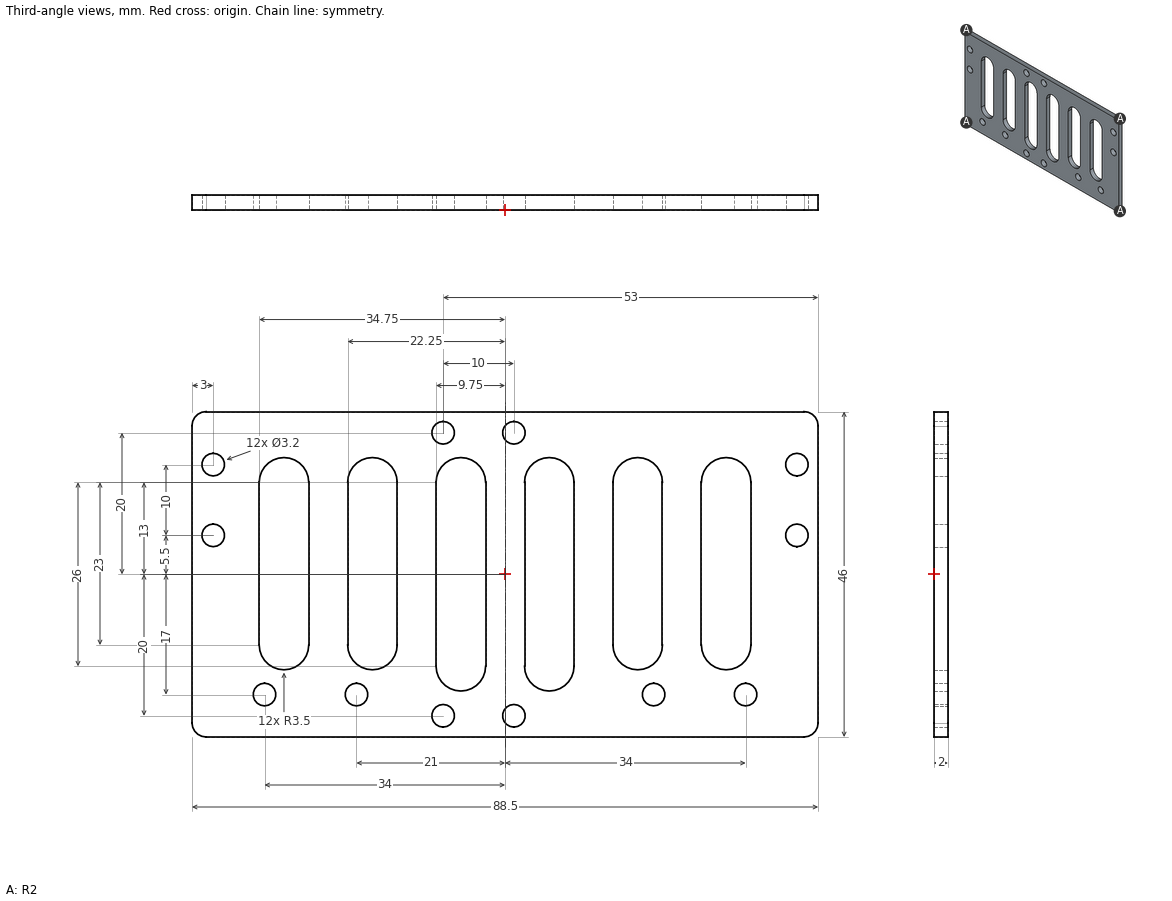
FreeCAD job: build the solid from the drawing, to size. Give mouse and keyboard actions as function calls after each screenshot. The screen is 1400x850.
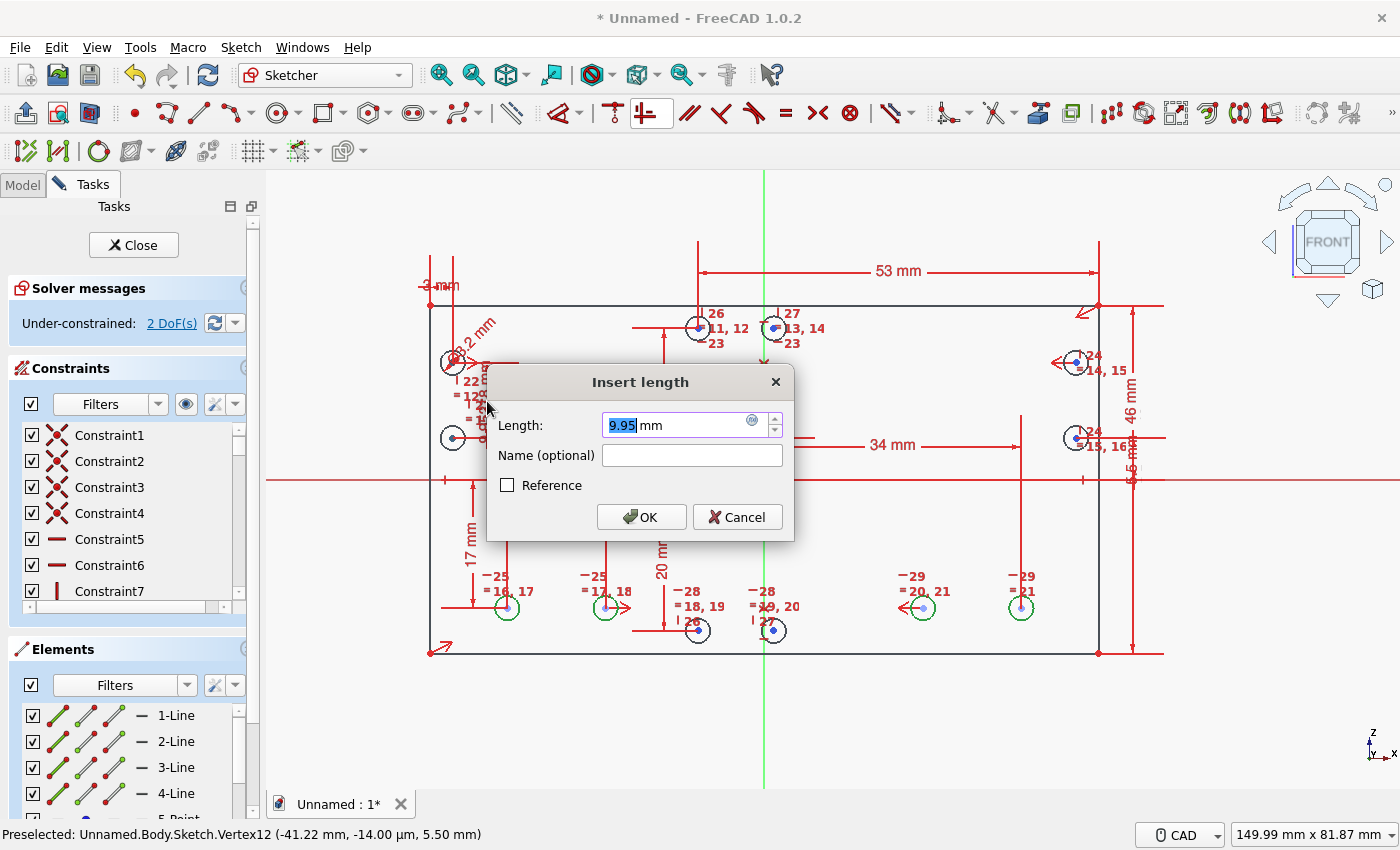
text(10)
key(Return)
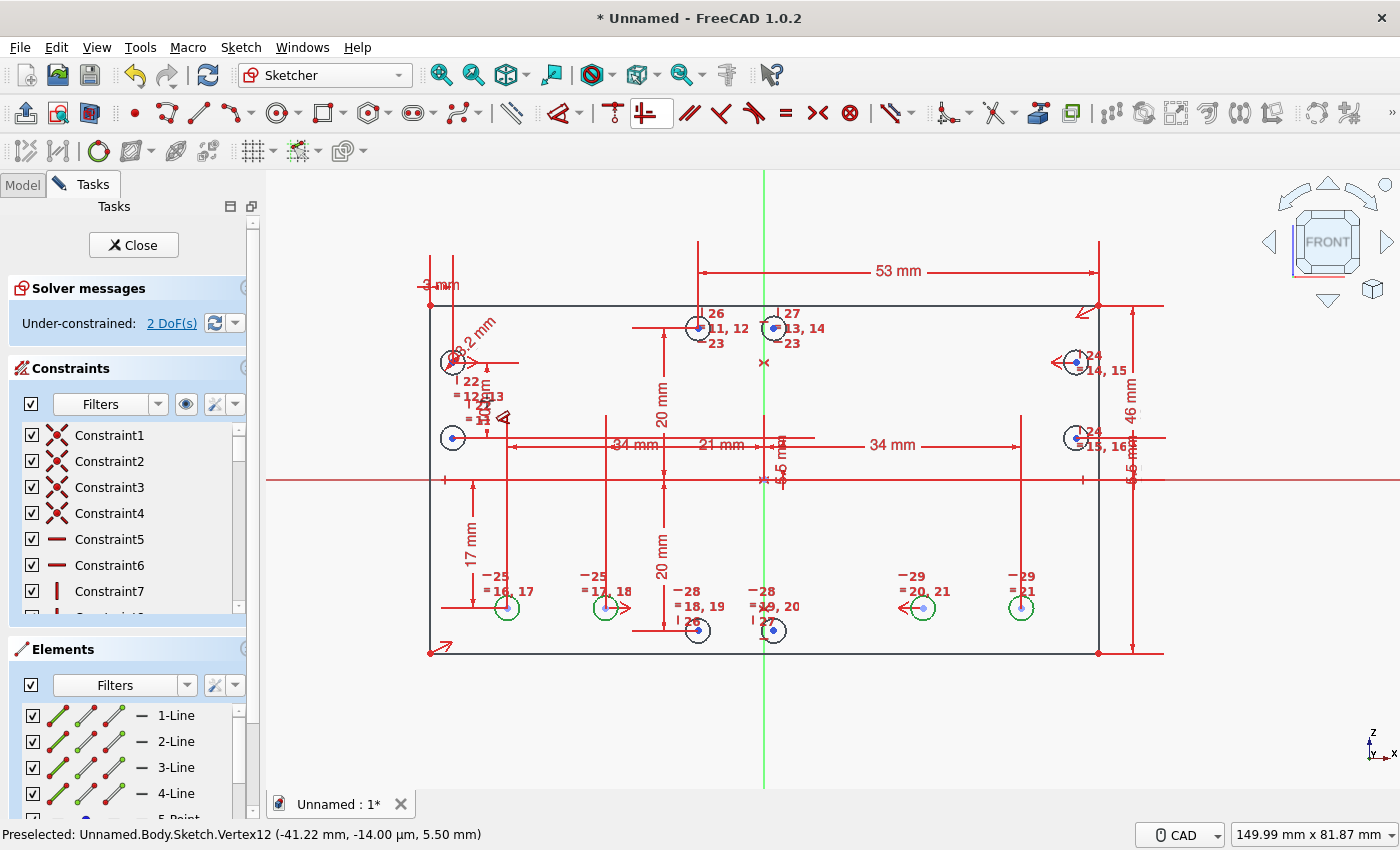
click(698, 328)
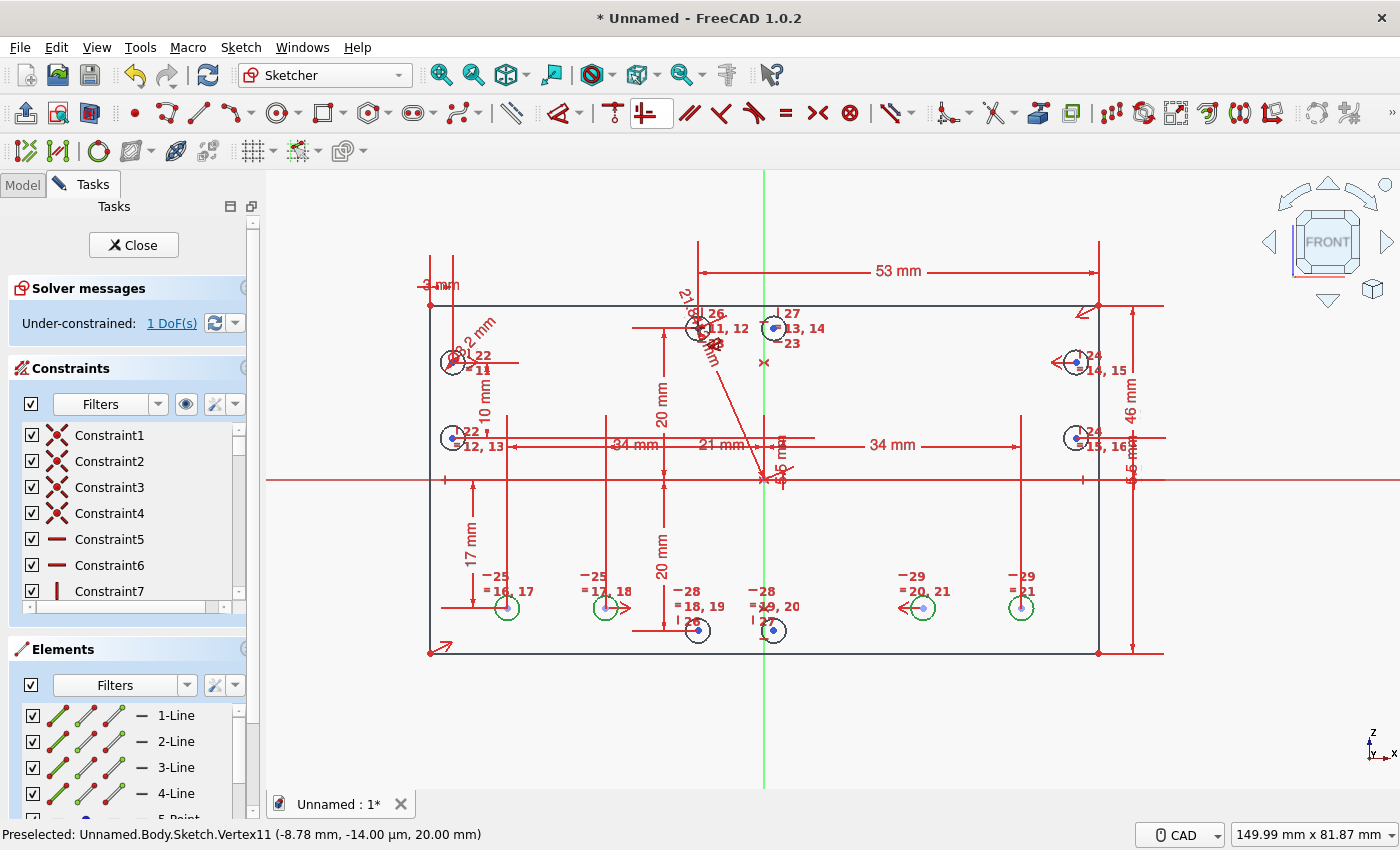
click(774, 328)
click(736, 362)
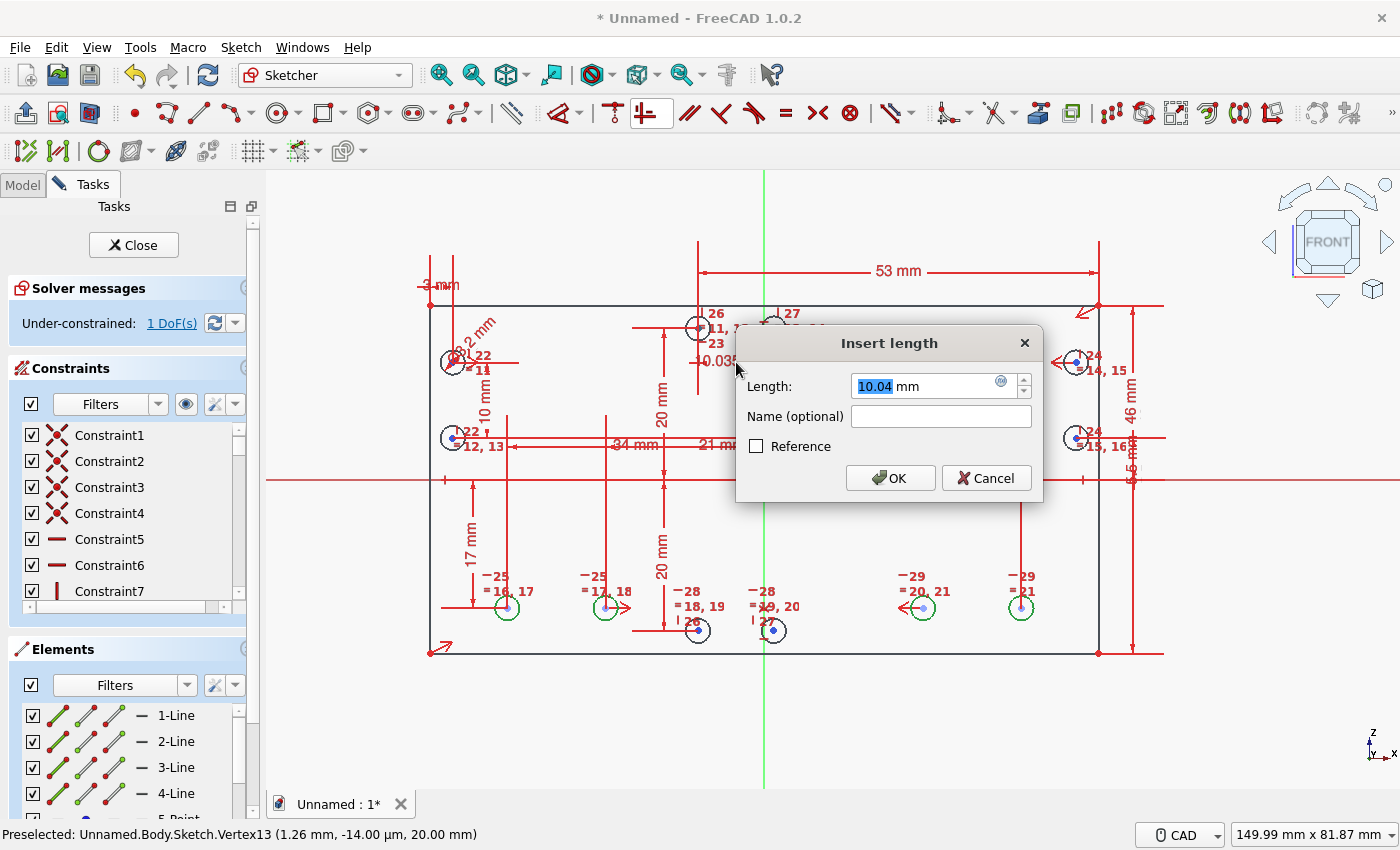
text(10)
key(Return)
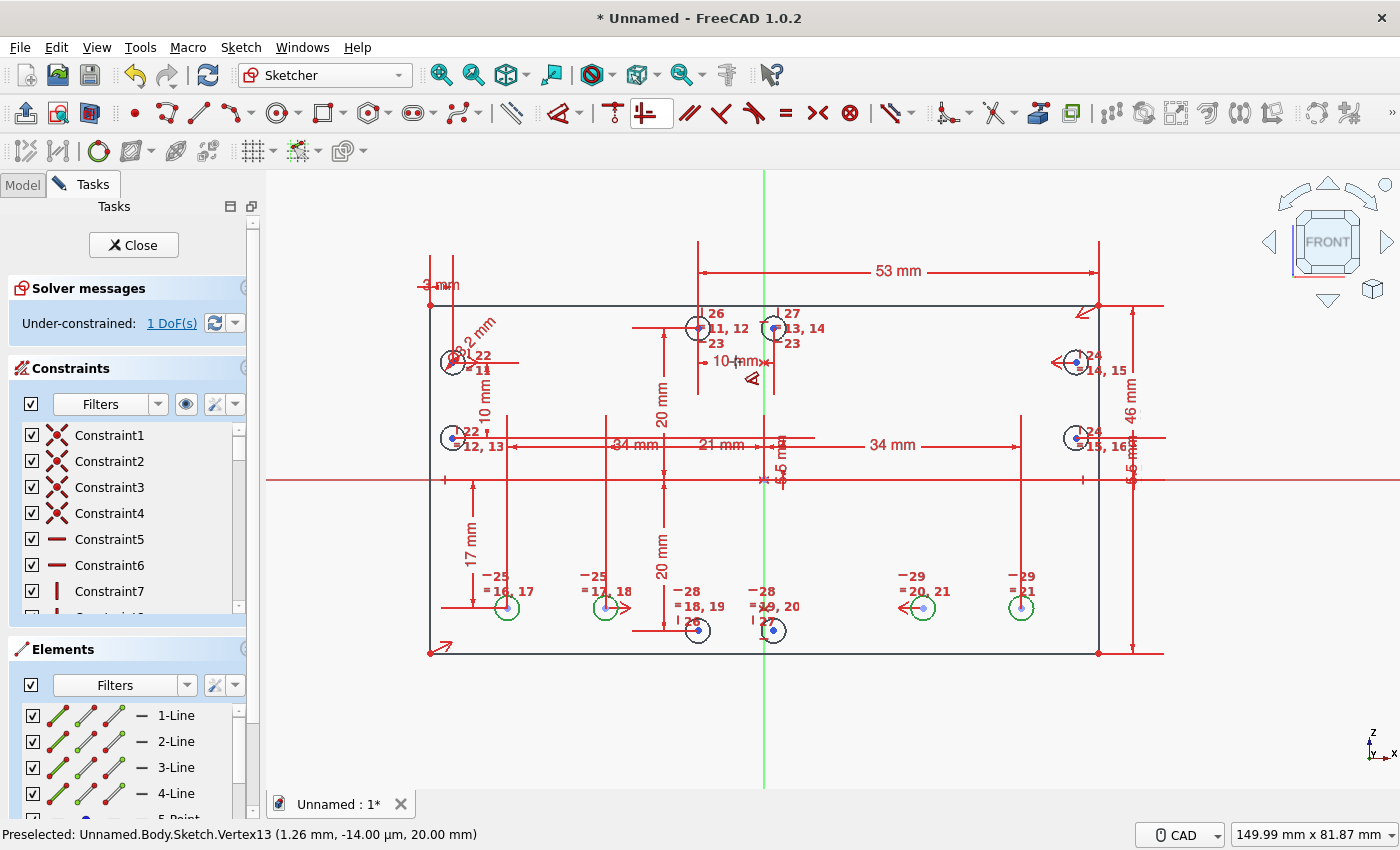
click(631, 654)
click(611, 688)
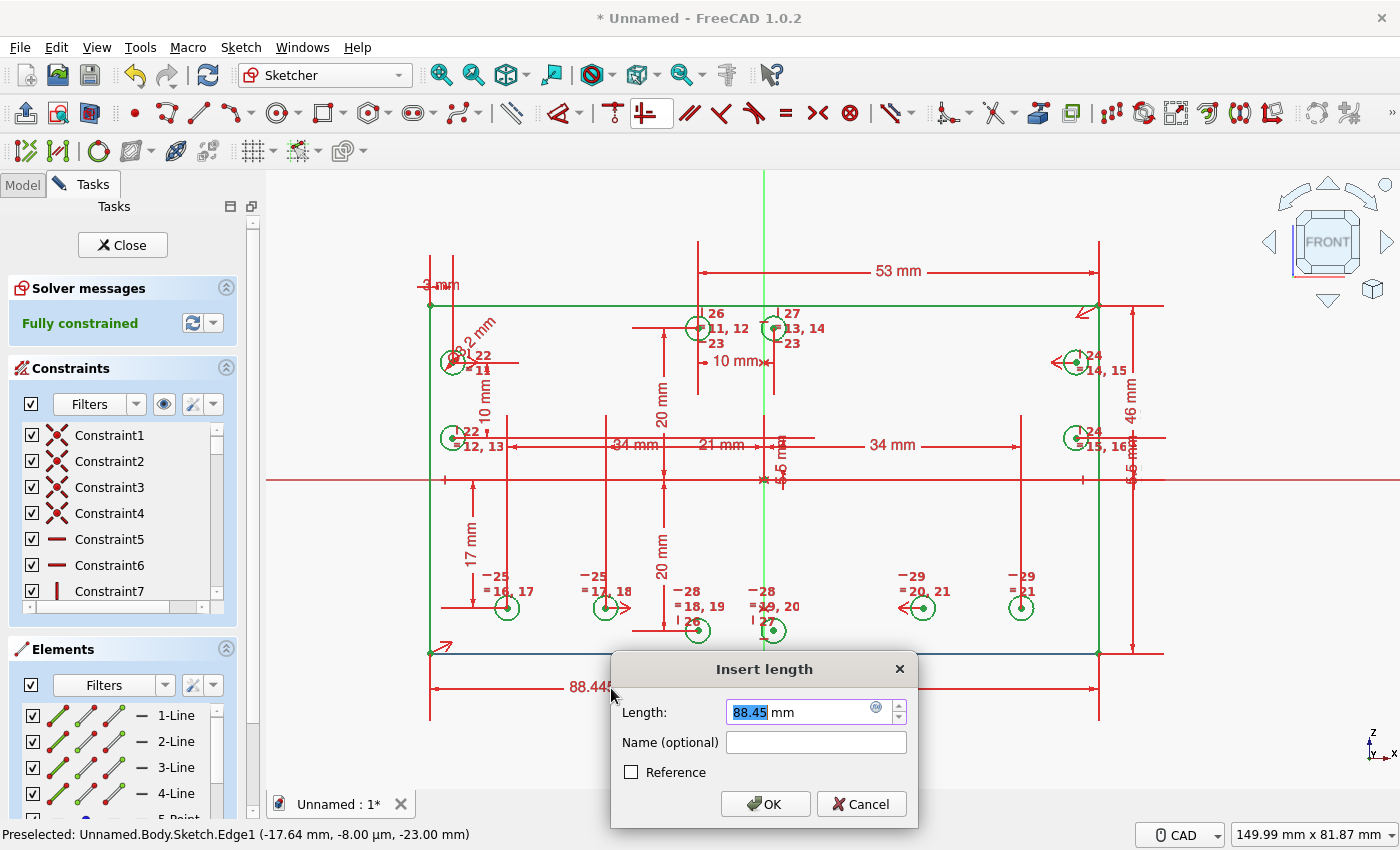
text(88.5)
key(Return)
key(Escape)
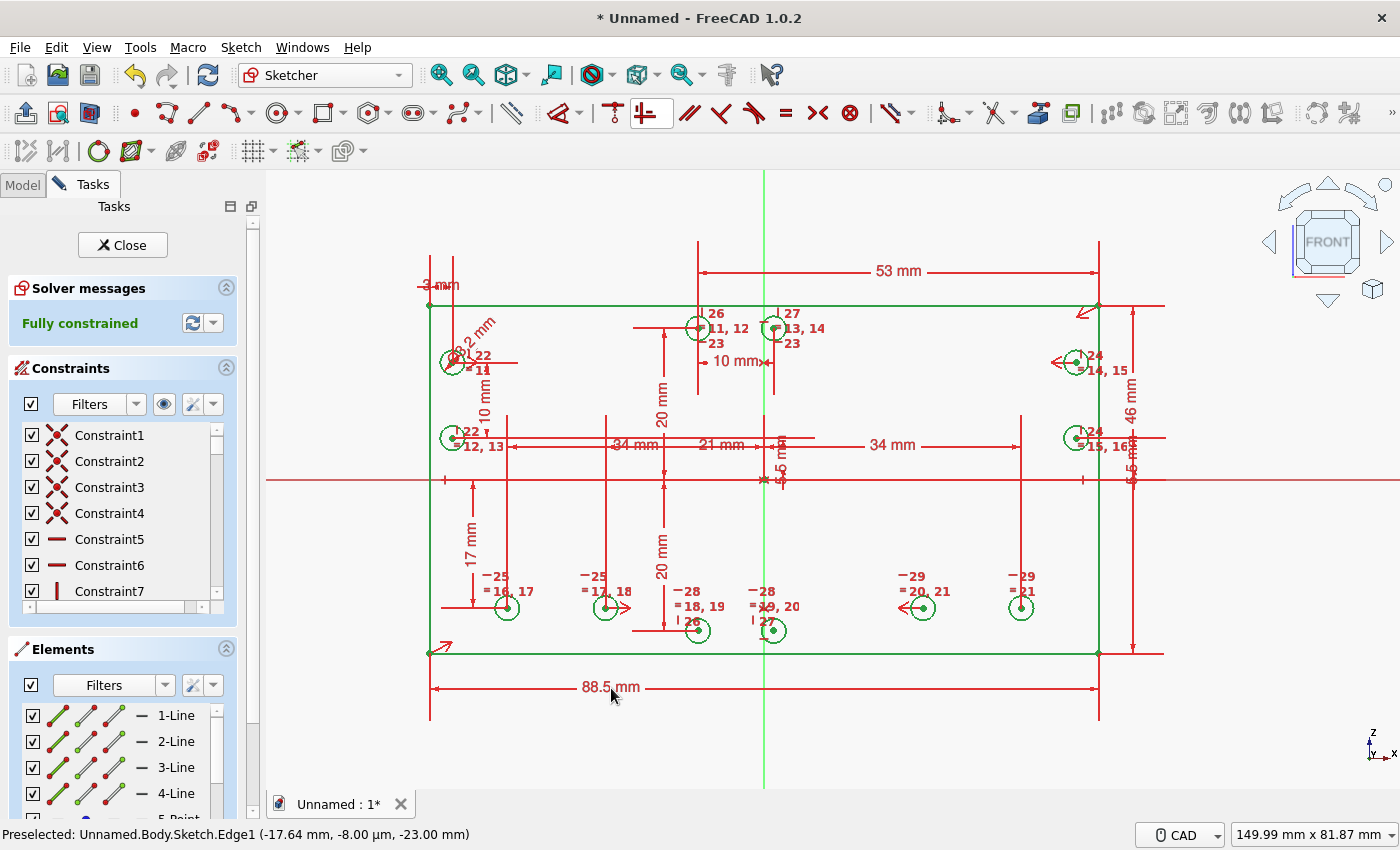
click(123, 245)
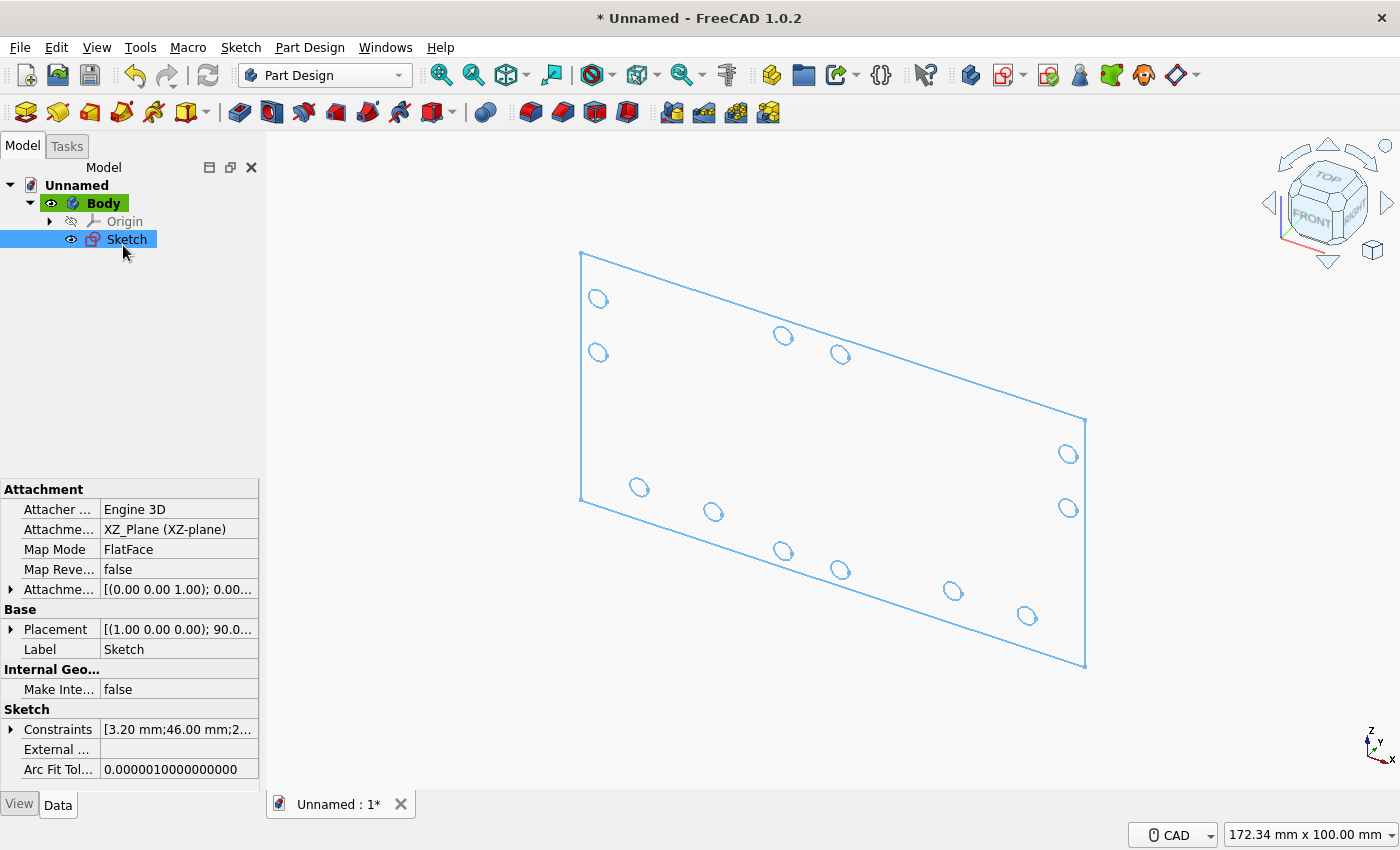
click(26, 112)